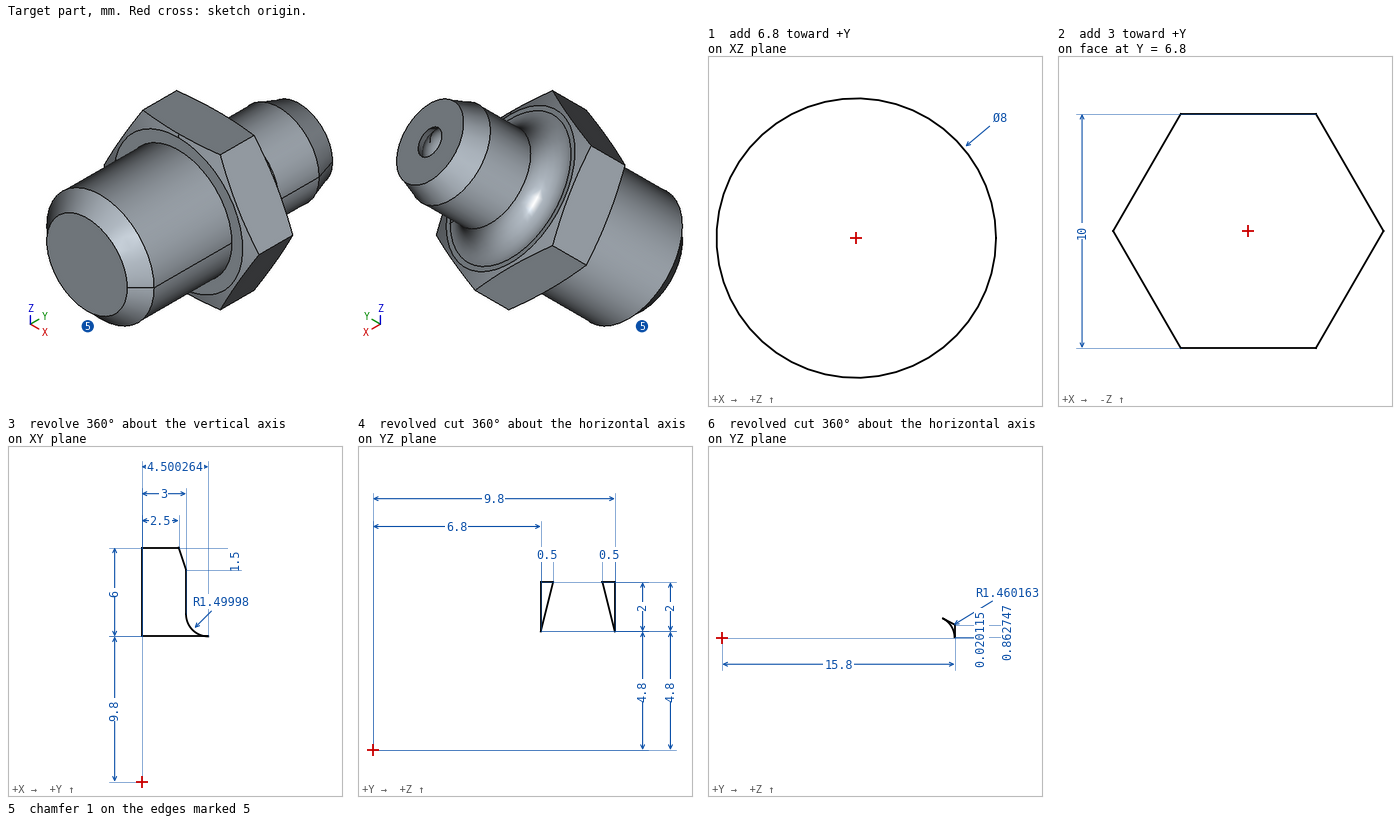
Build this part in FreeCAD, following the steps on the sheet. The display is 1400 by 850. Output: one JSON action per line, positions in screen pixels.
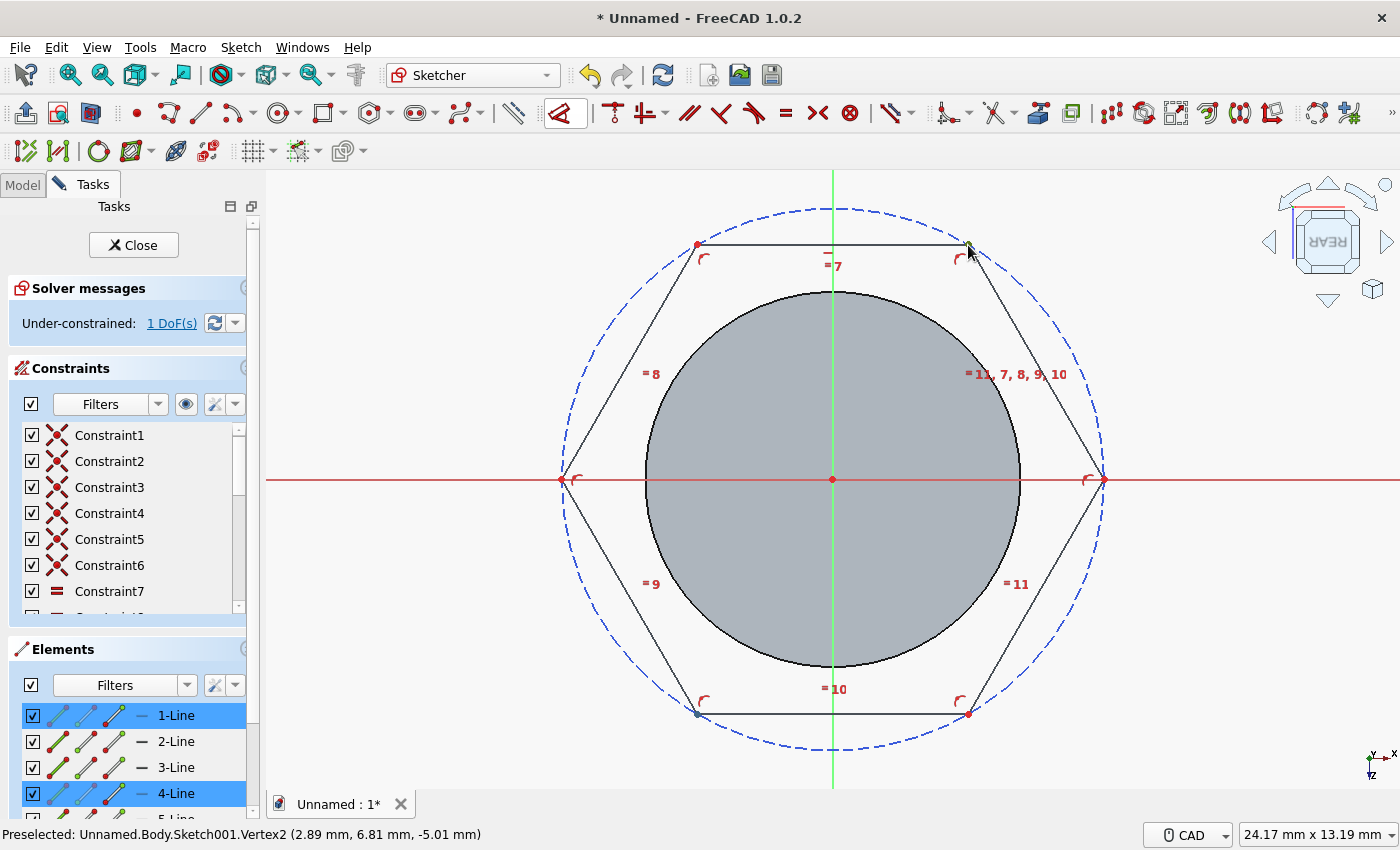
{"action": "key", "text": "i"}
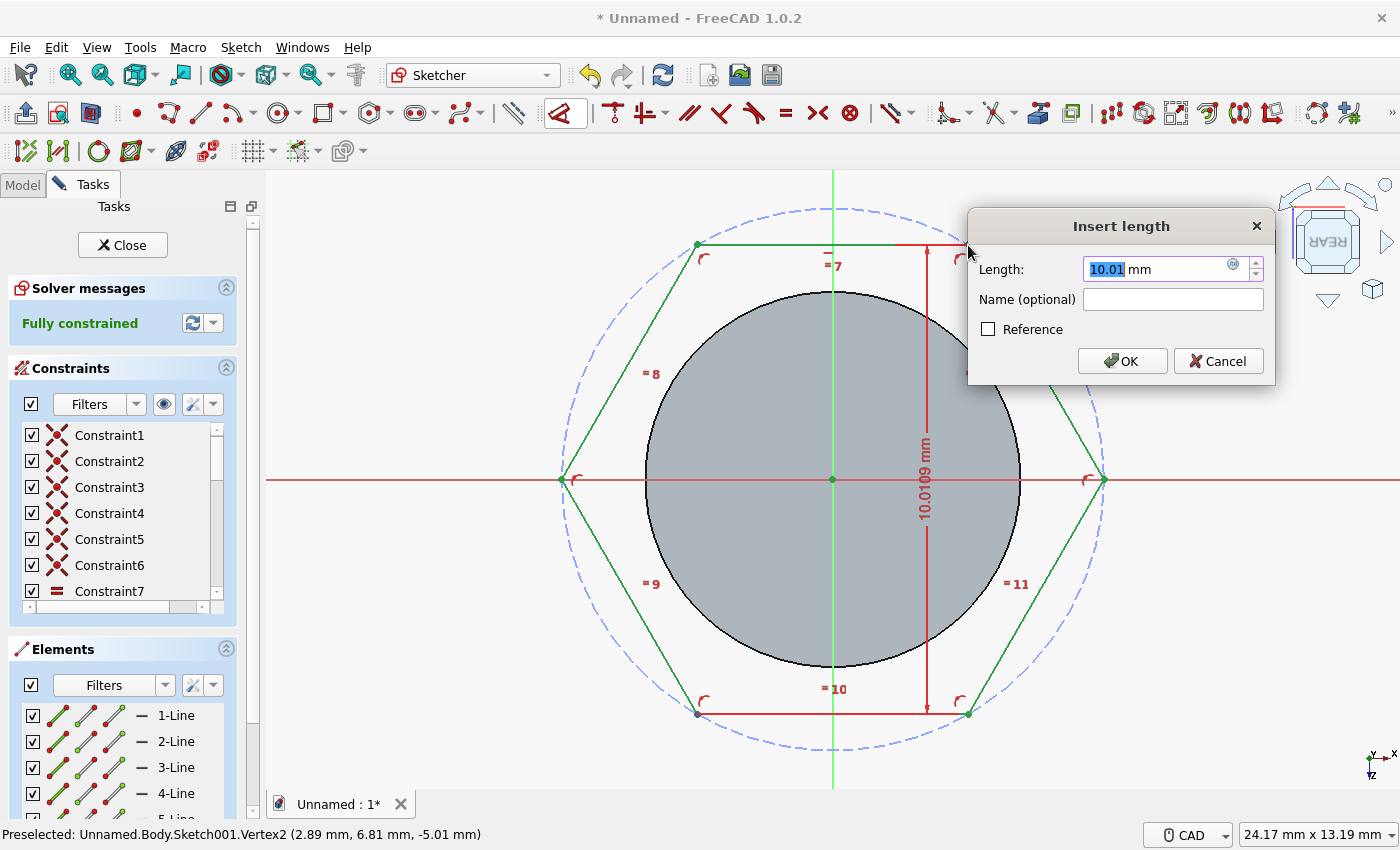
{"action": "type", "text": "10"}
{"action": "key", "text": "Return"}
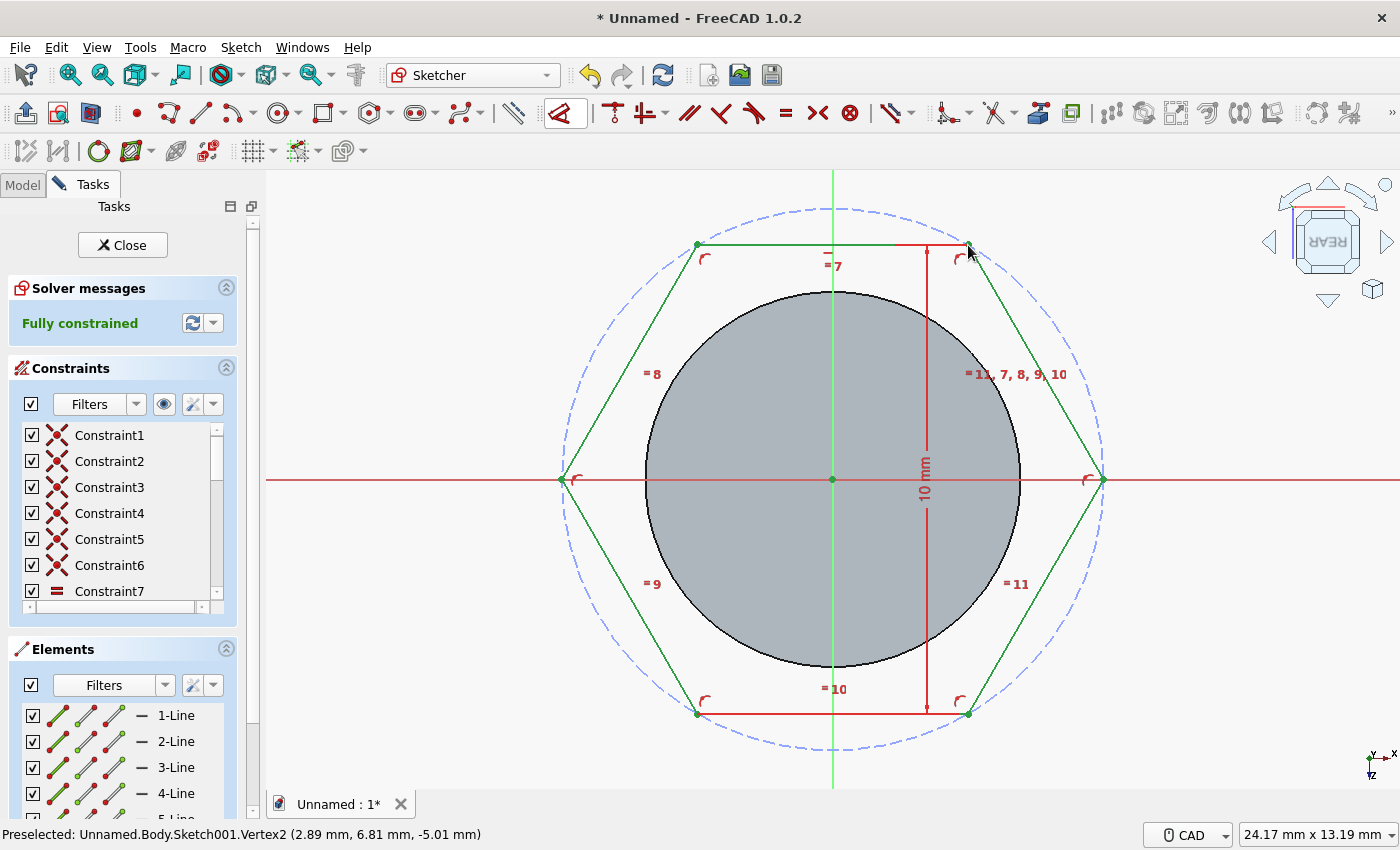
{"action": "left_click", "coordinate": [123, 245]}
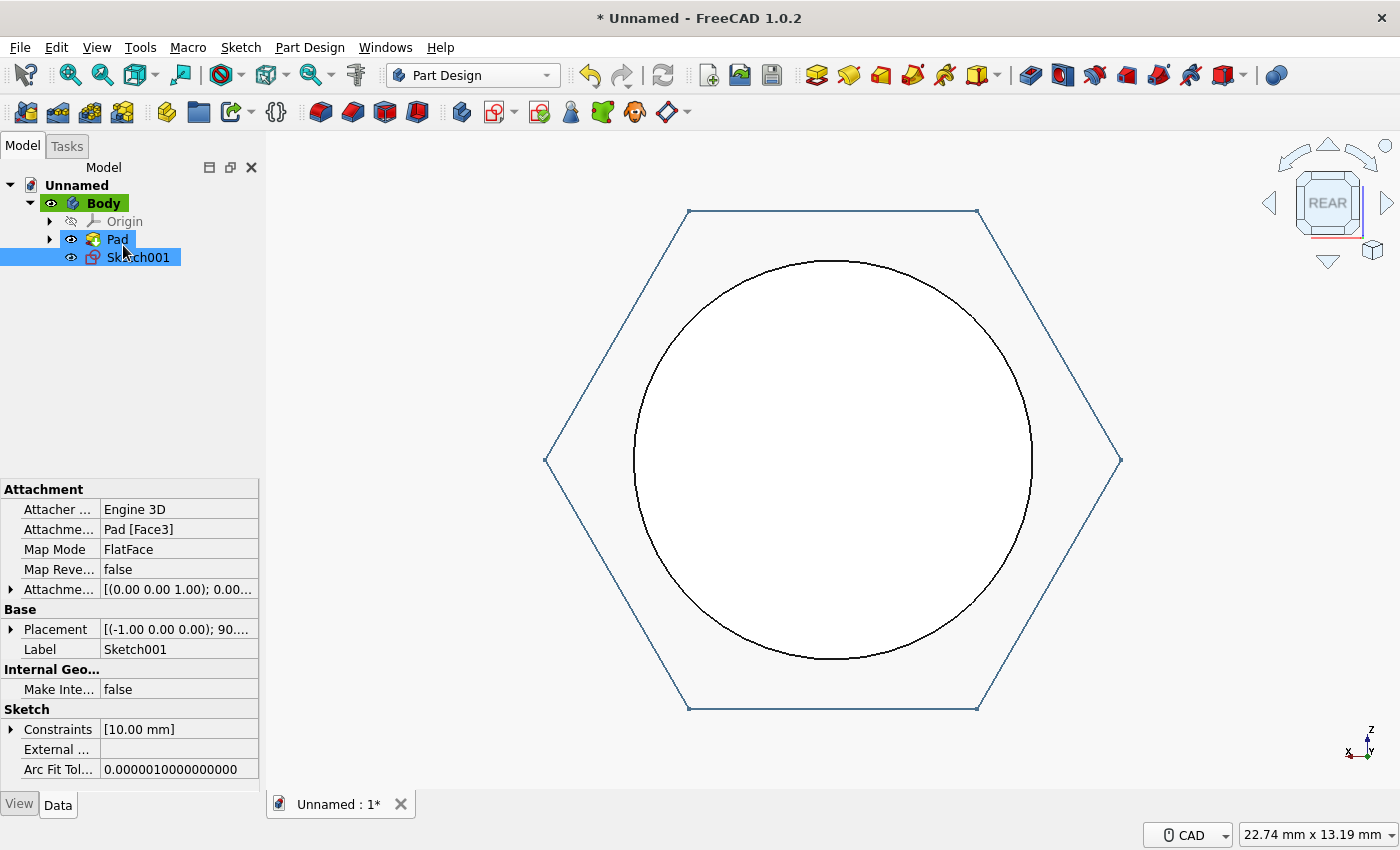
{"action": "left_click", "coordinate": [818, 76]}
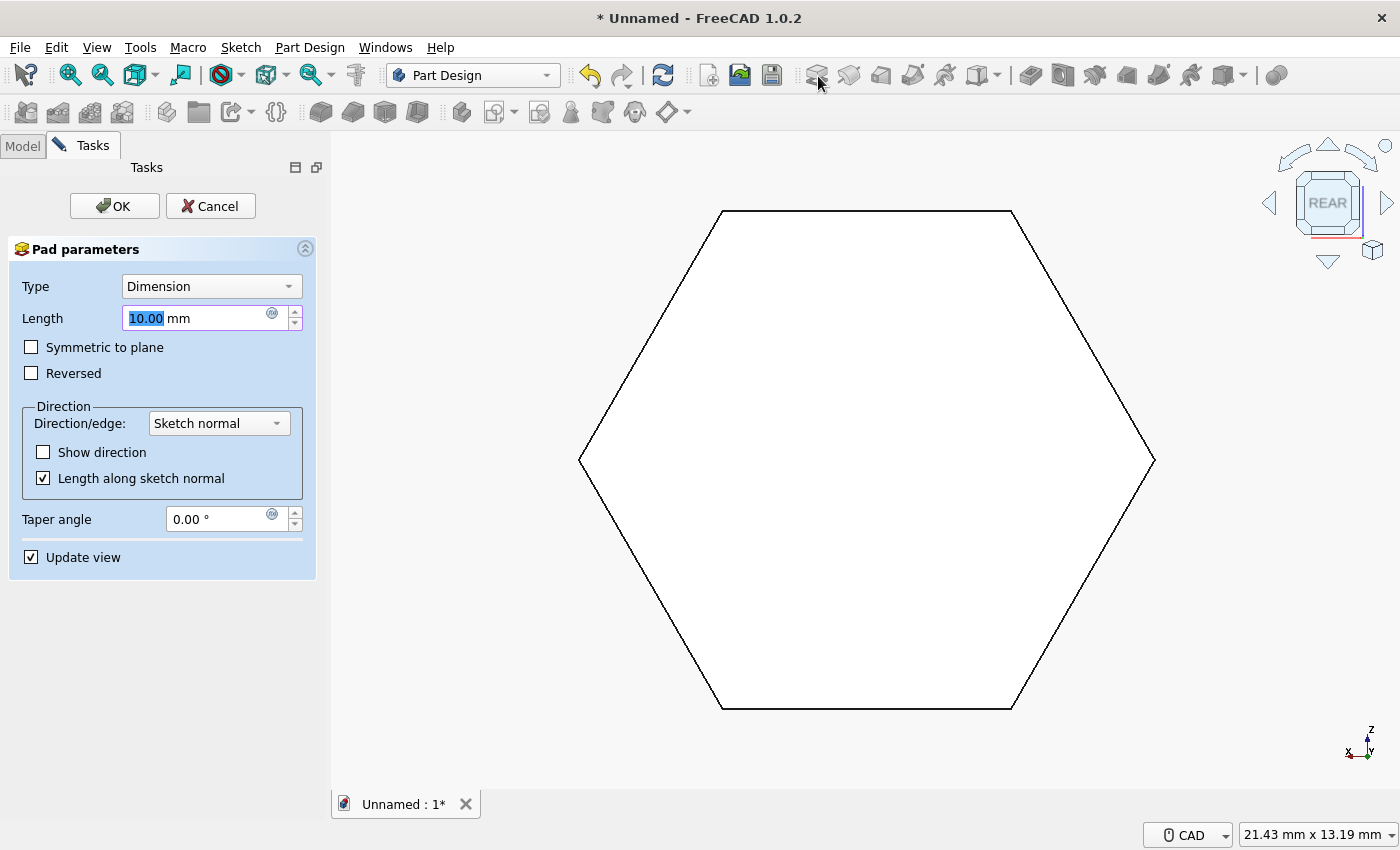
{"action": "type", "text": "3"}
{"action": "key", "text": "Tab"}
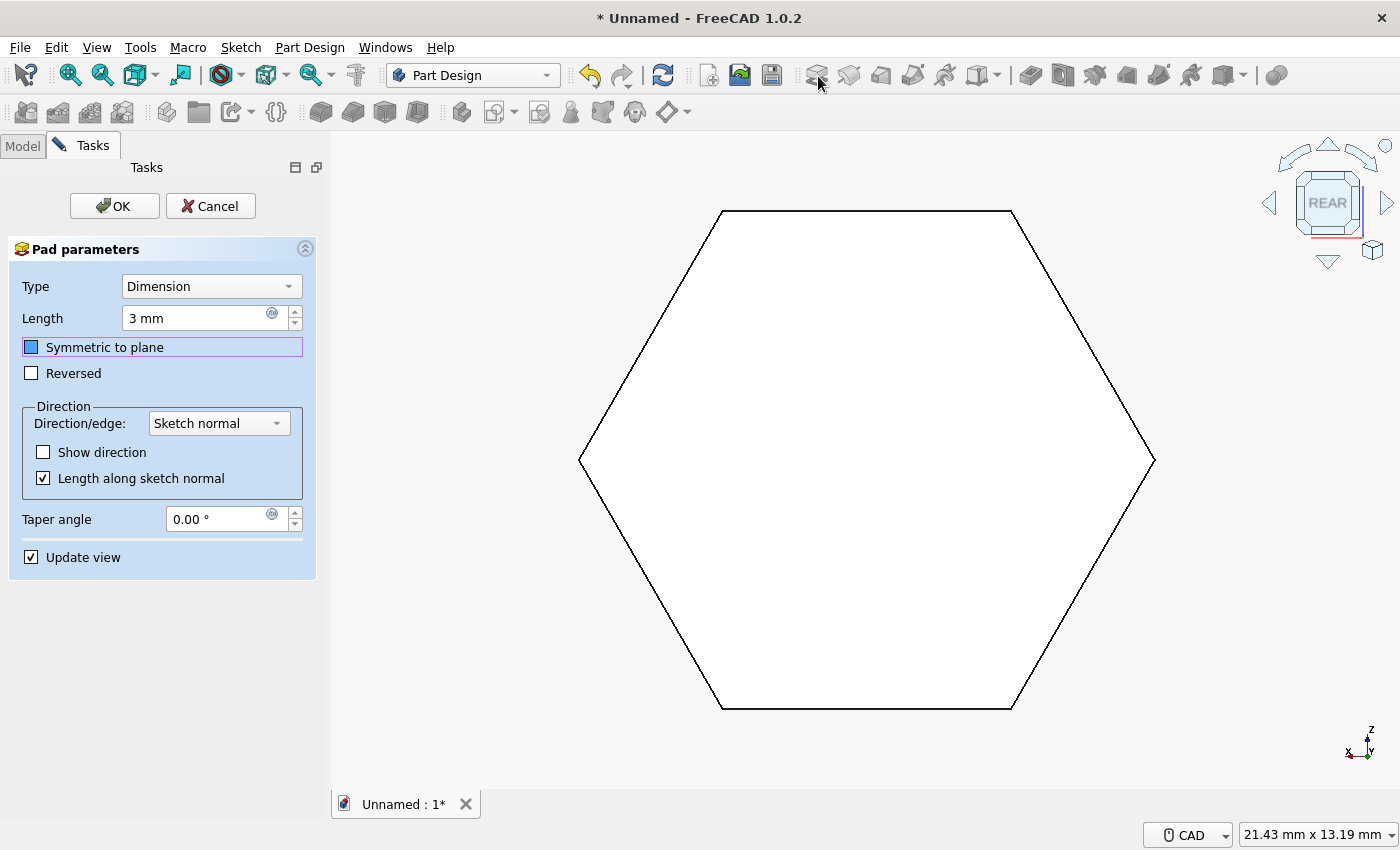
{"action": "left_click", "coordinate": [115, 206]}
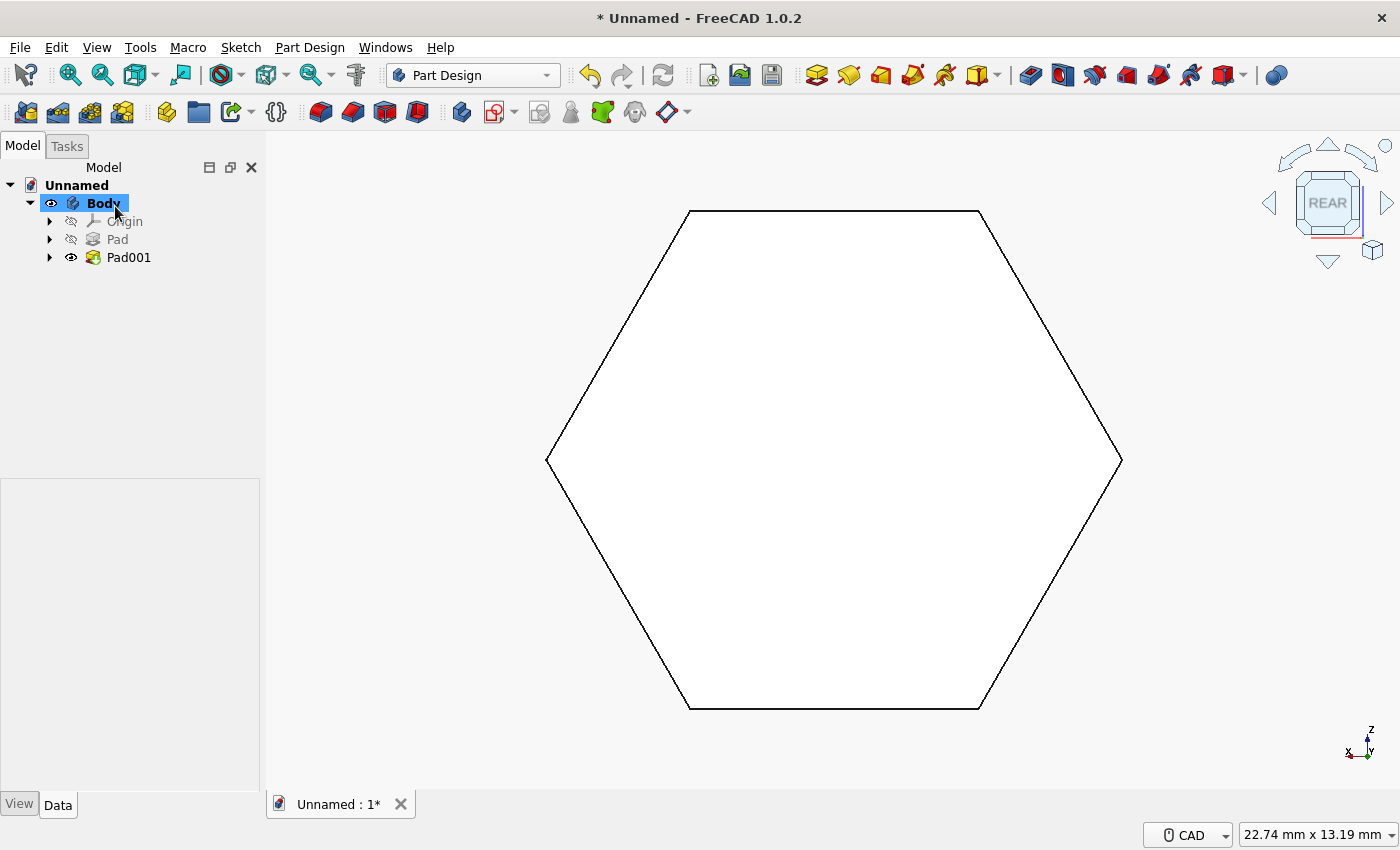
{"action": "left_click", "coordinate": [494, 112]}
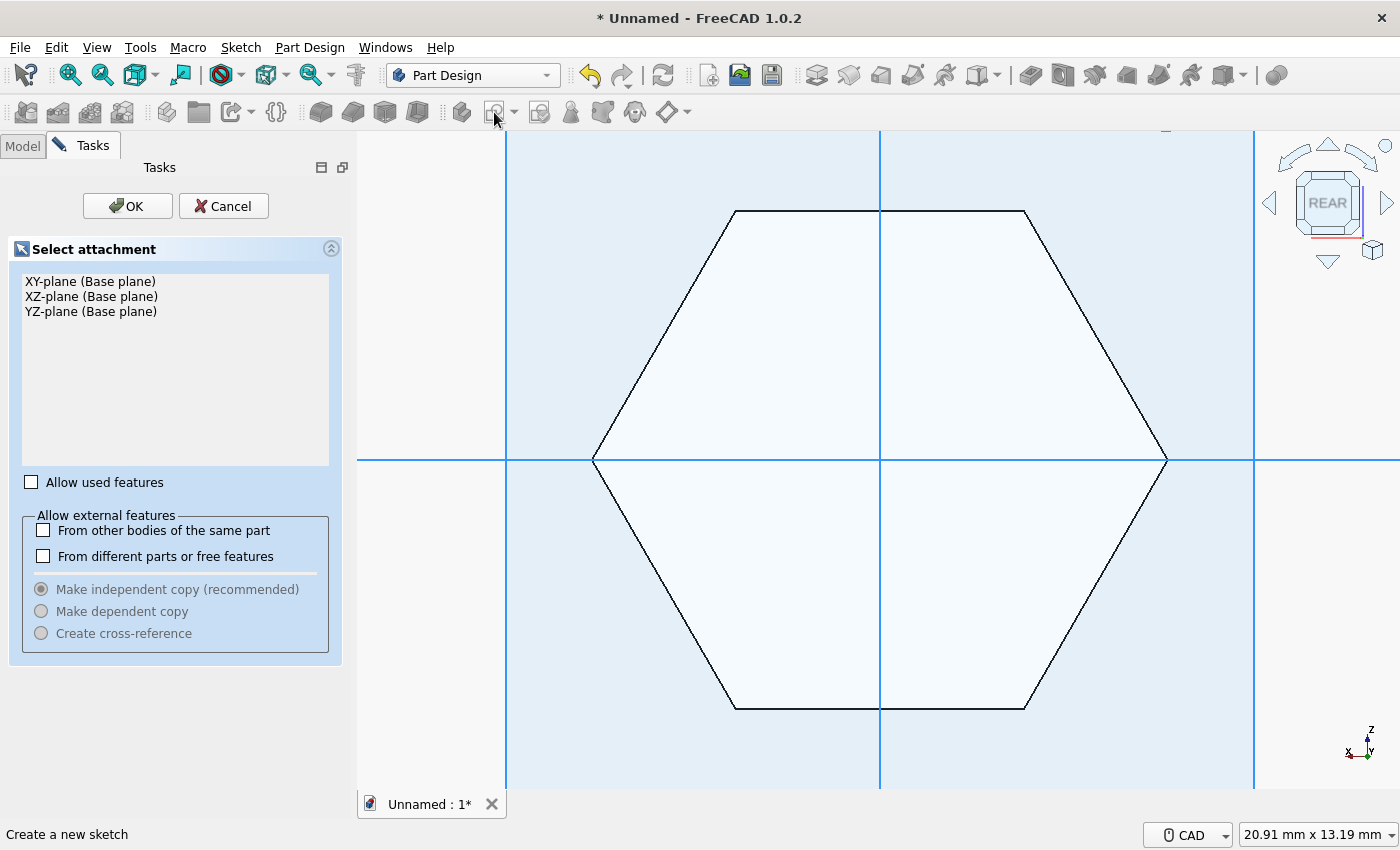
{"action": "left_click", "coordinate": [82, 282]}